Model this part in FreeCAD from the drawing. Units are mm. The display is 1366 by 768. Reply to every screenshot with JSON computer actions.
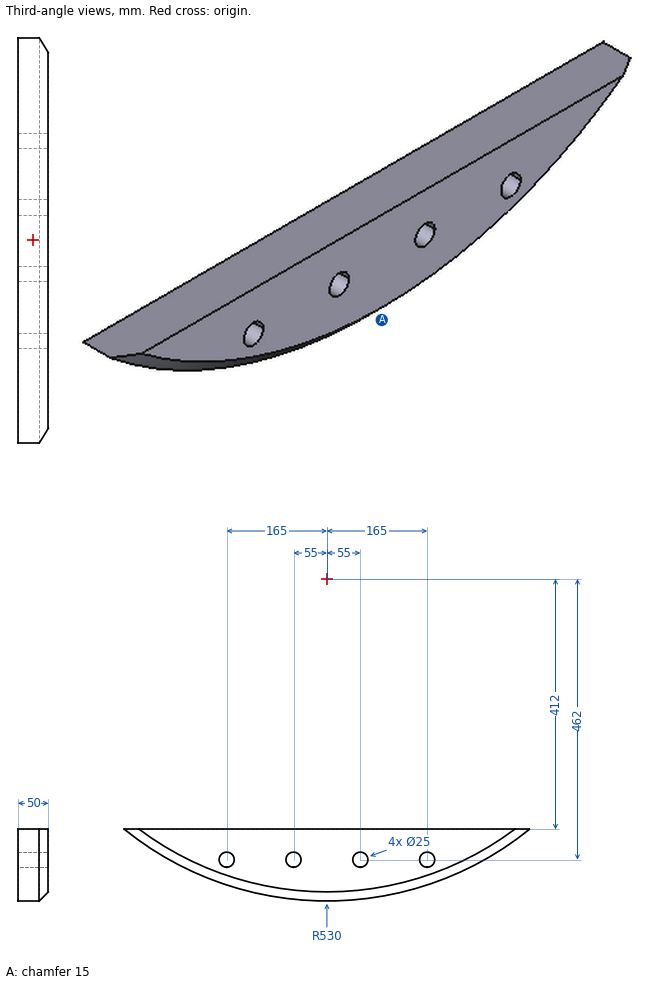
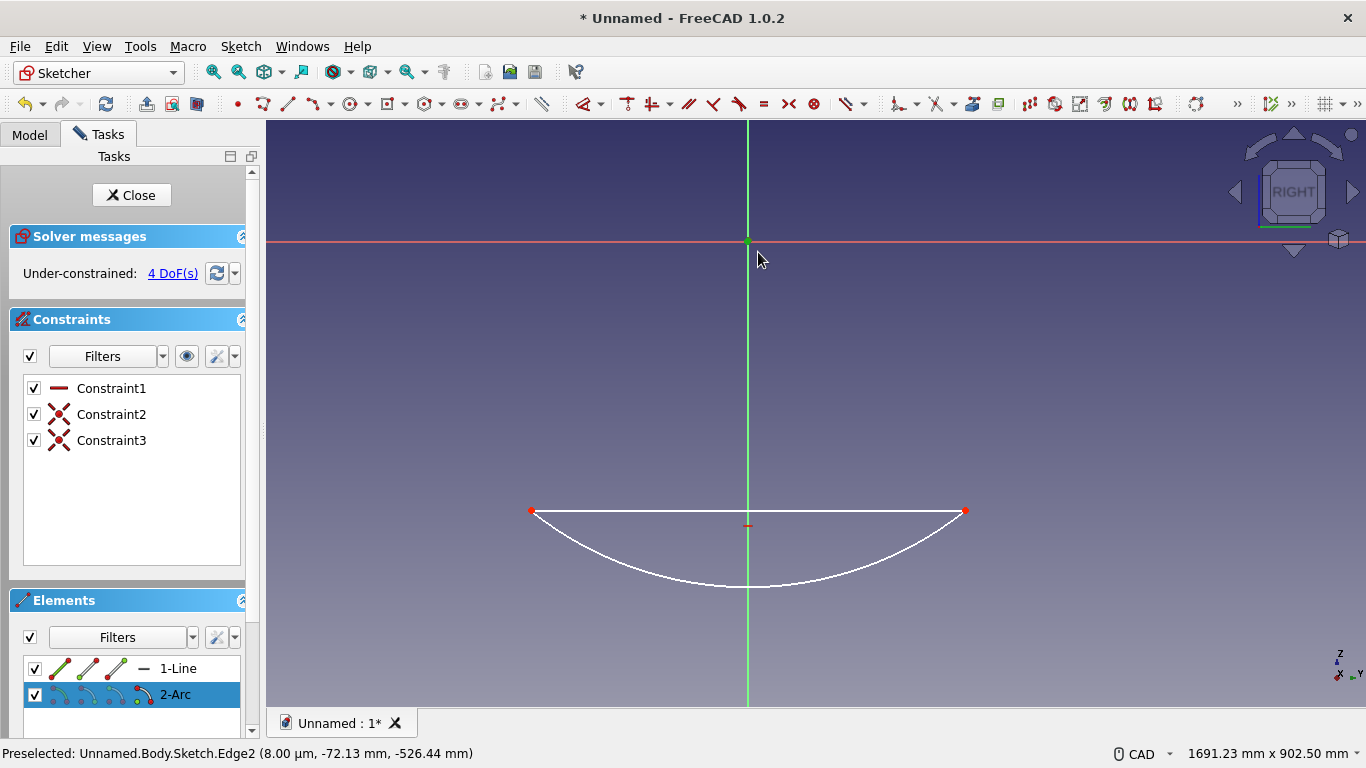
{"action": "left_click", "coordinate": [627, 104]}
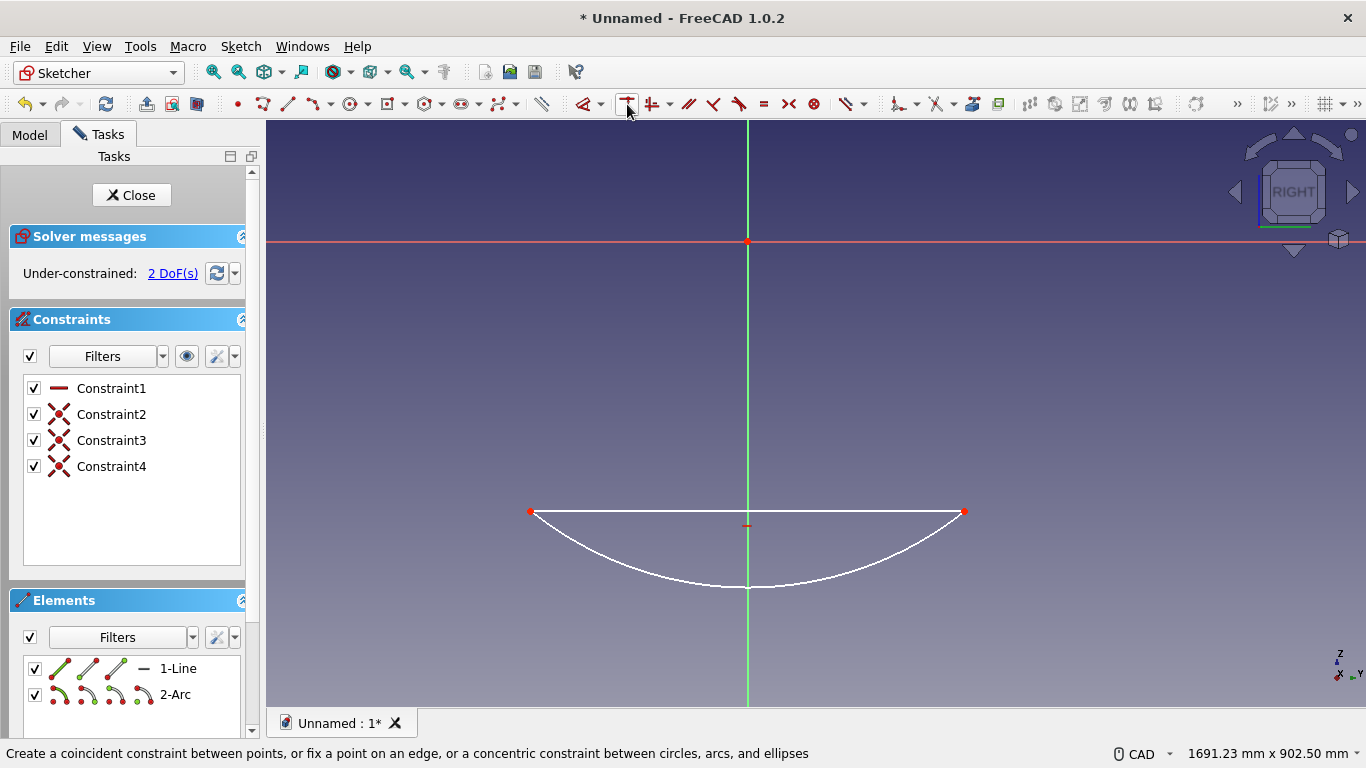
{"action": "left_click", "coordinate": [582, 104]}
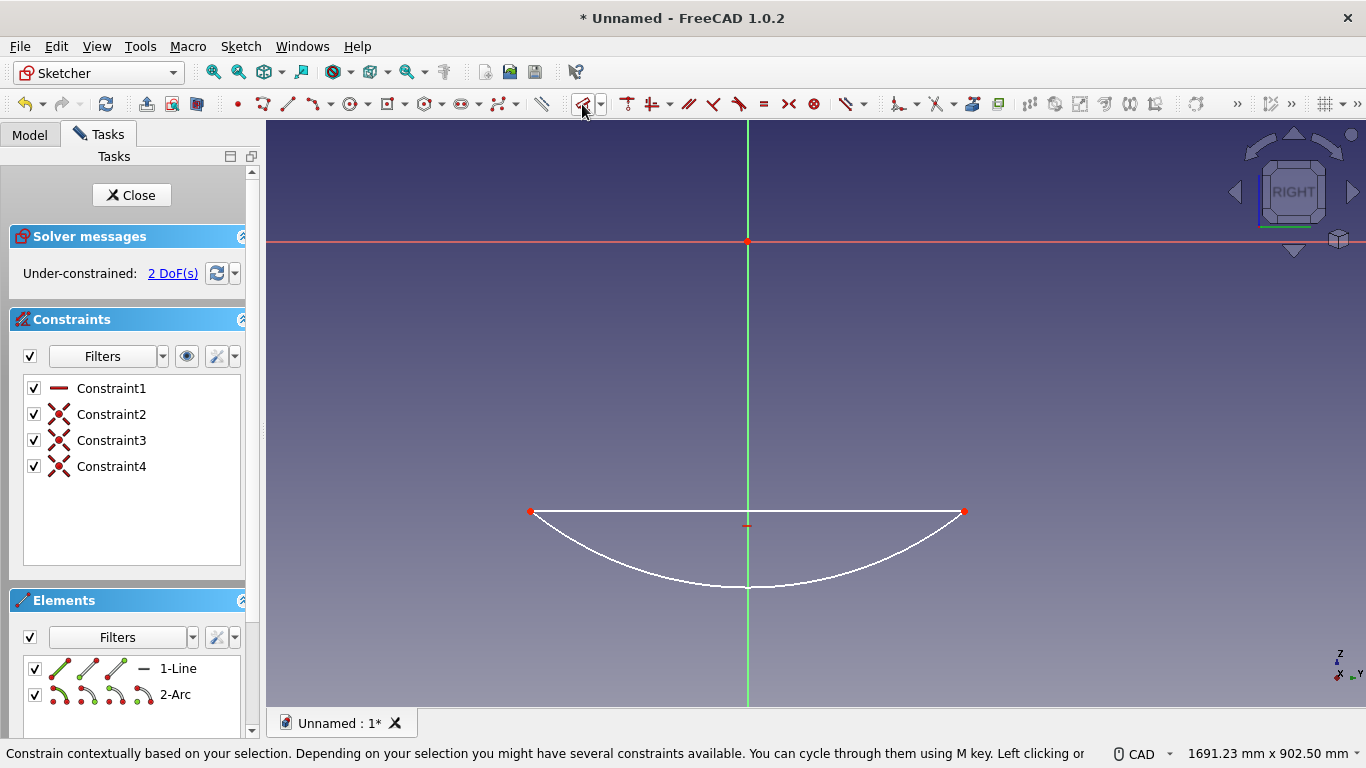
{"action": "left_click", "coordinate": [655, 575]}
{"action": "left_click", "coordinate": [646, 606]}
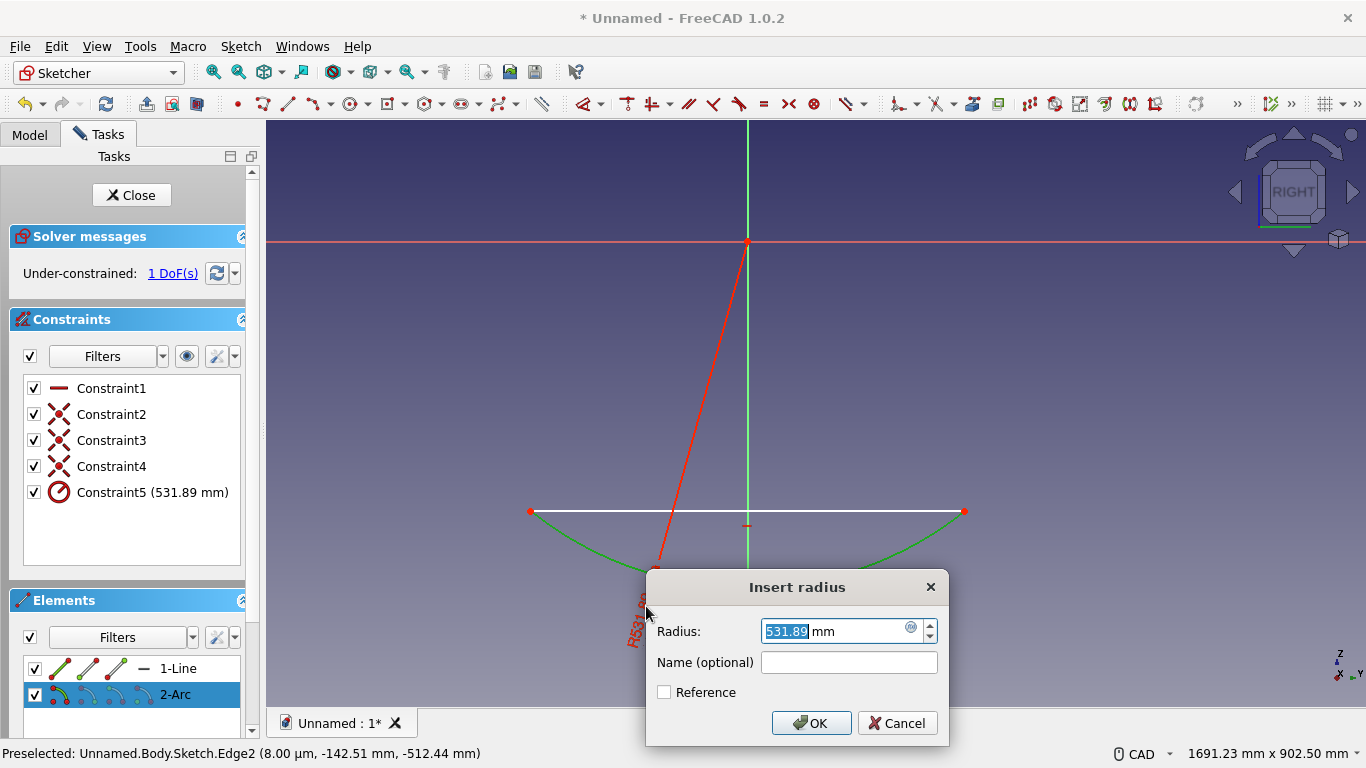
{"action": "type", "text": "530"}
{"action": "key", "text": "Return"}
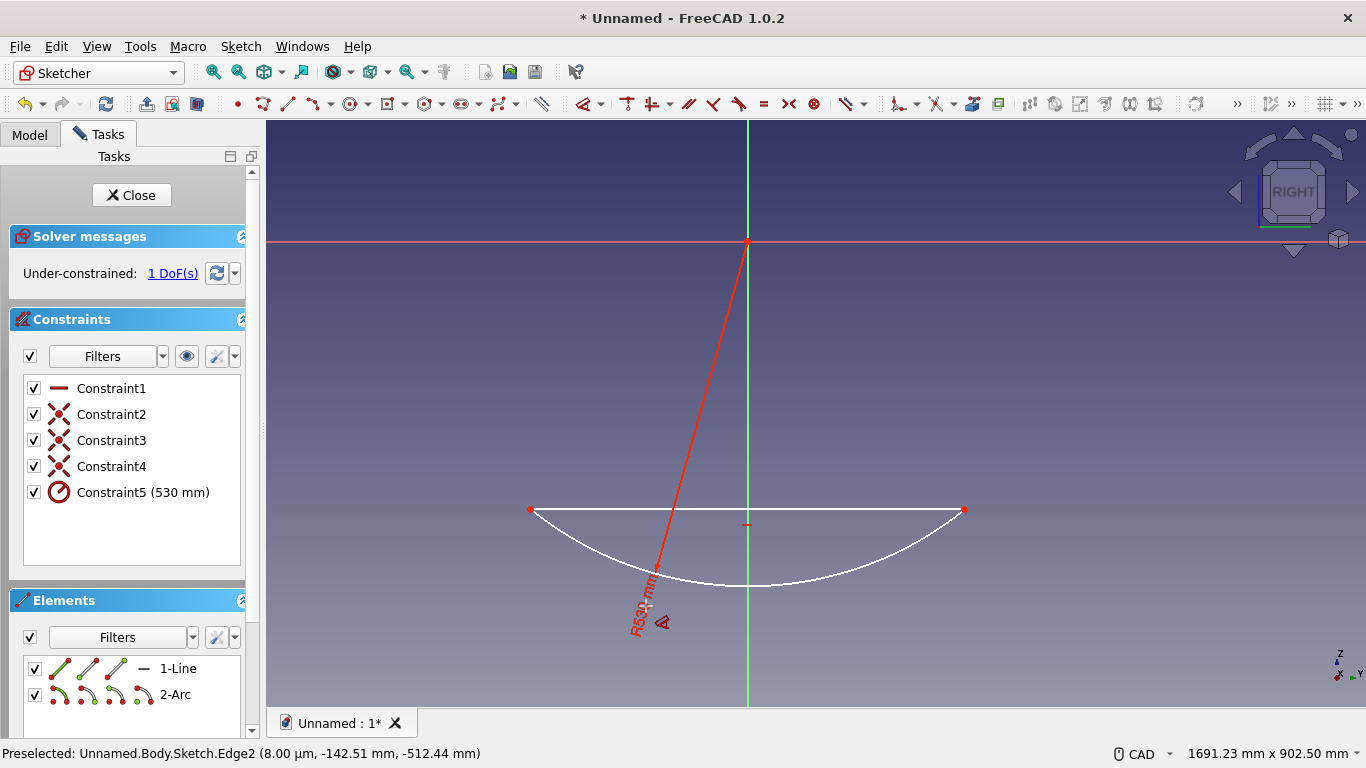
{"action": "left_click", "coordinate": [965, 509]}
{"action": "left_click", "coordinate": [999, 376]}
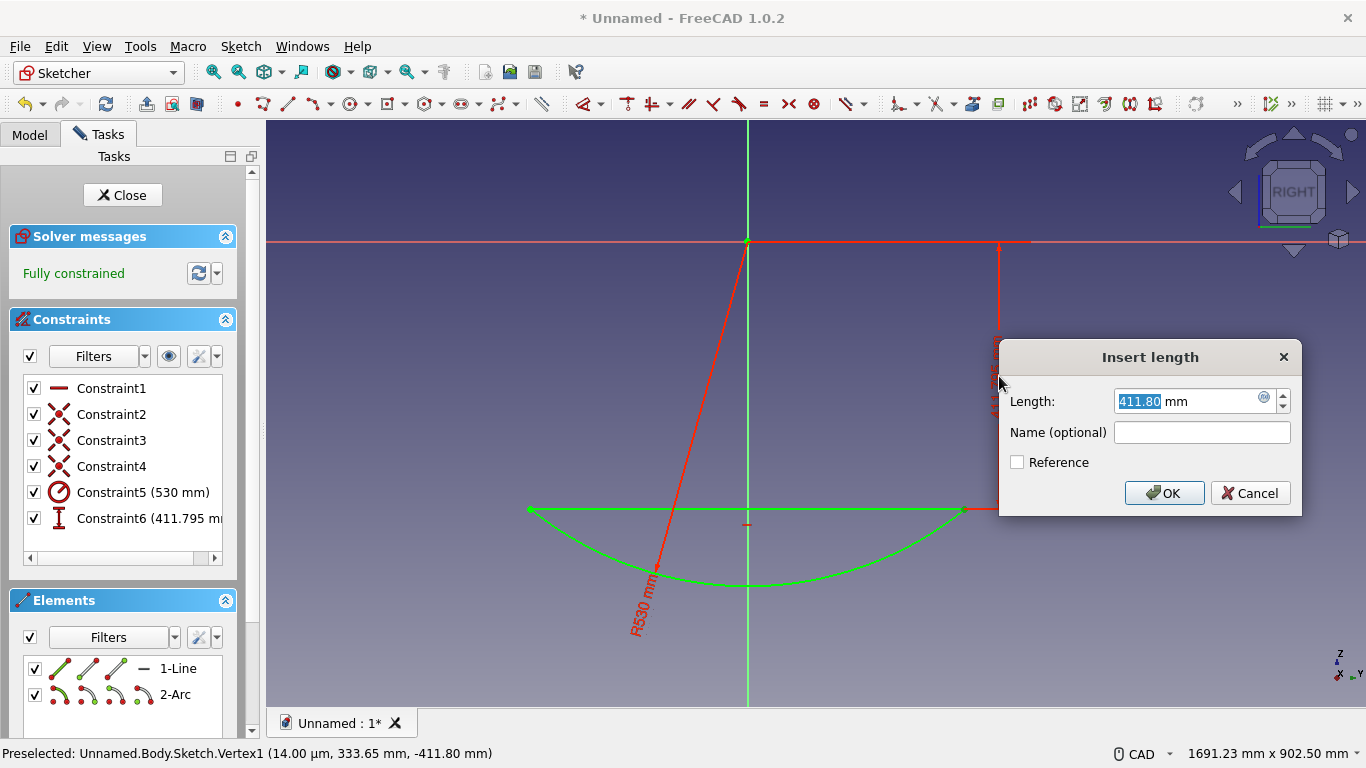
{"action": "type", "text": "412"}
{"action": "key", "text": "Return"}
{"action": "key", "text": "Escape"}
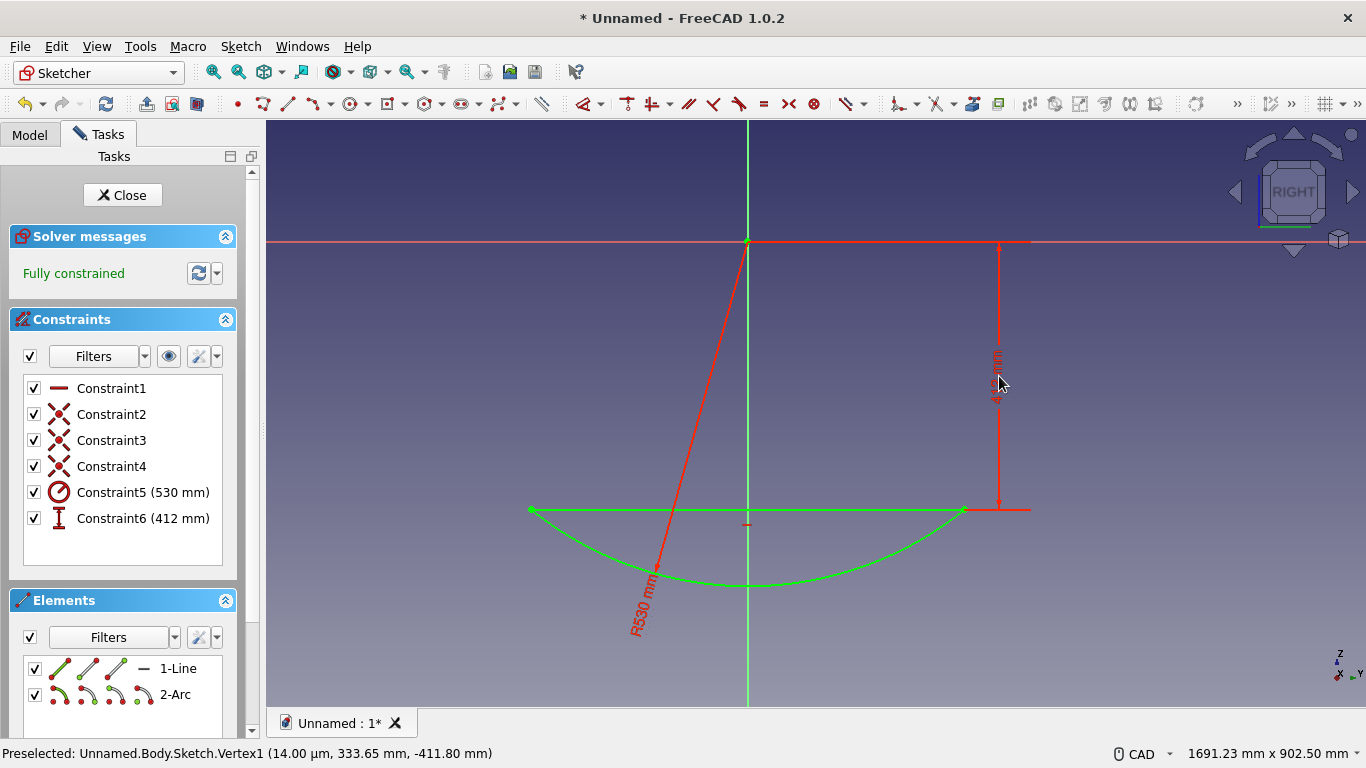
{"action": "left_click", "coordinate": [123, 195]}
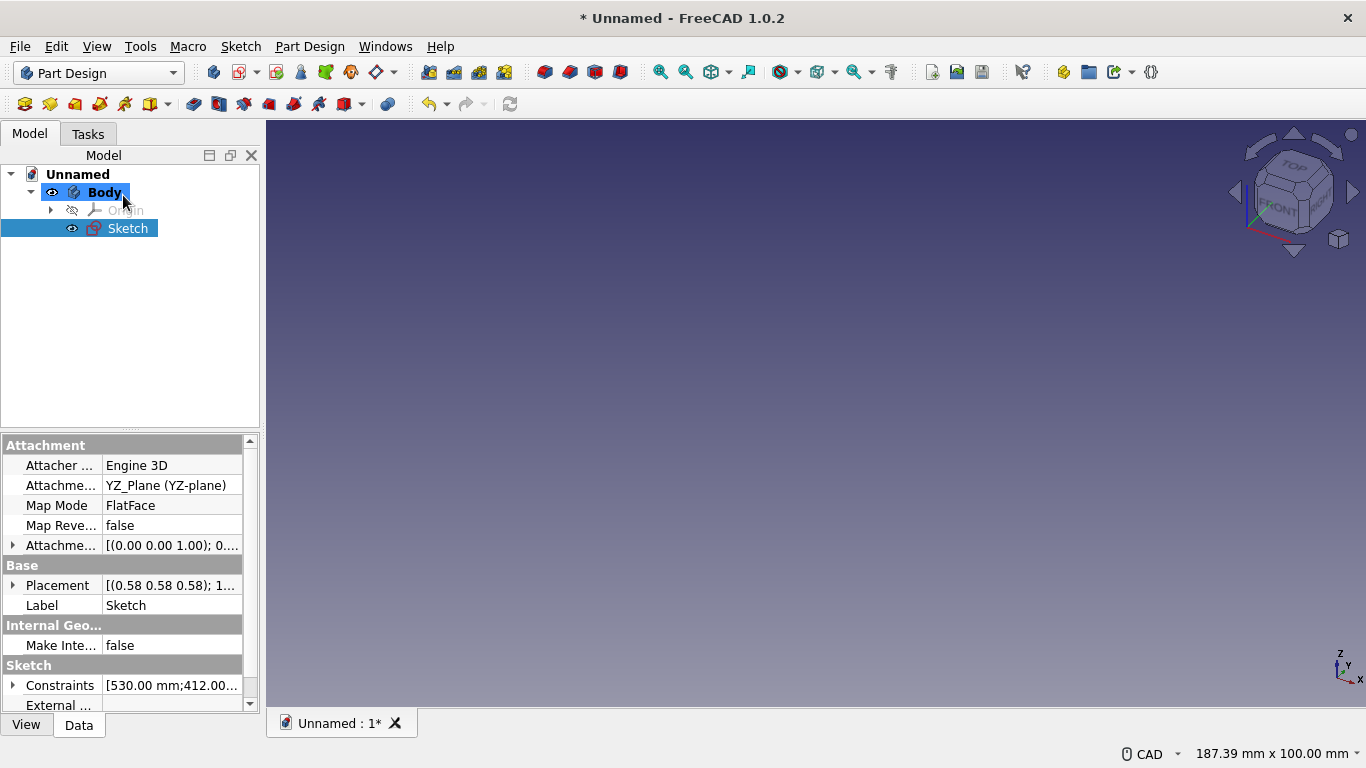
{"action": "left_click", "coordinate": [25, 104]}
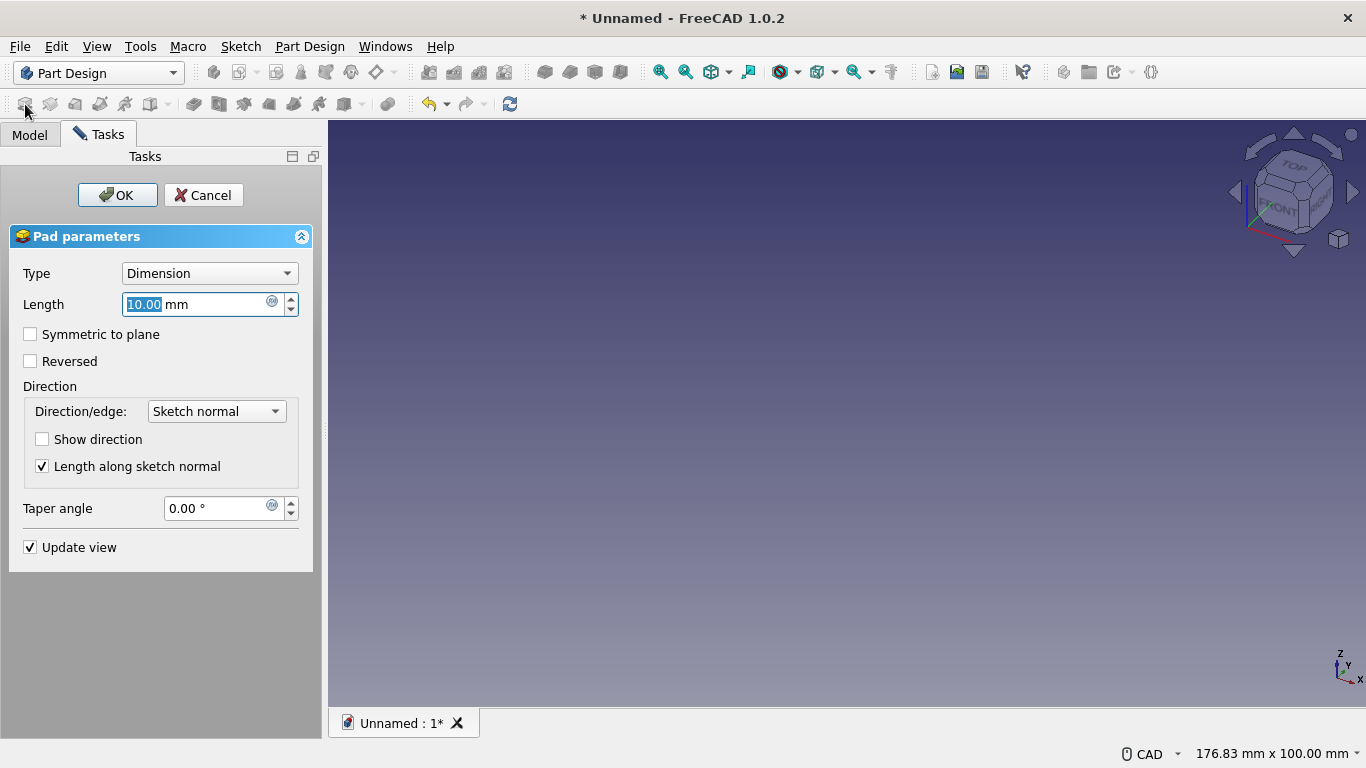
{"action": "type", "text": "50"}
{"action": "key", "text": "Tab"}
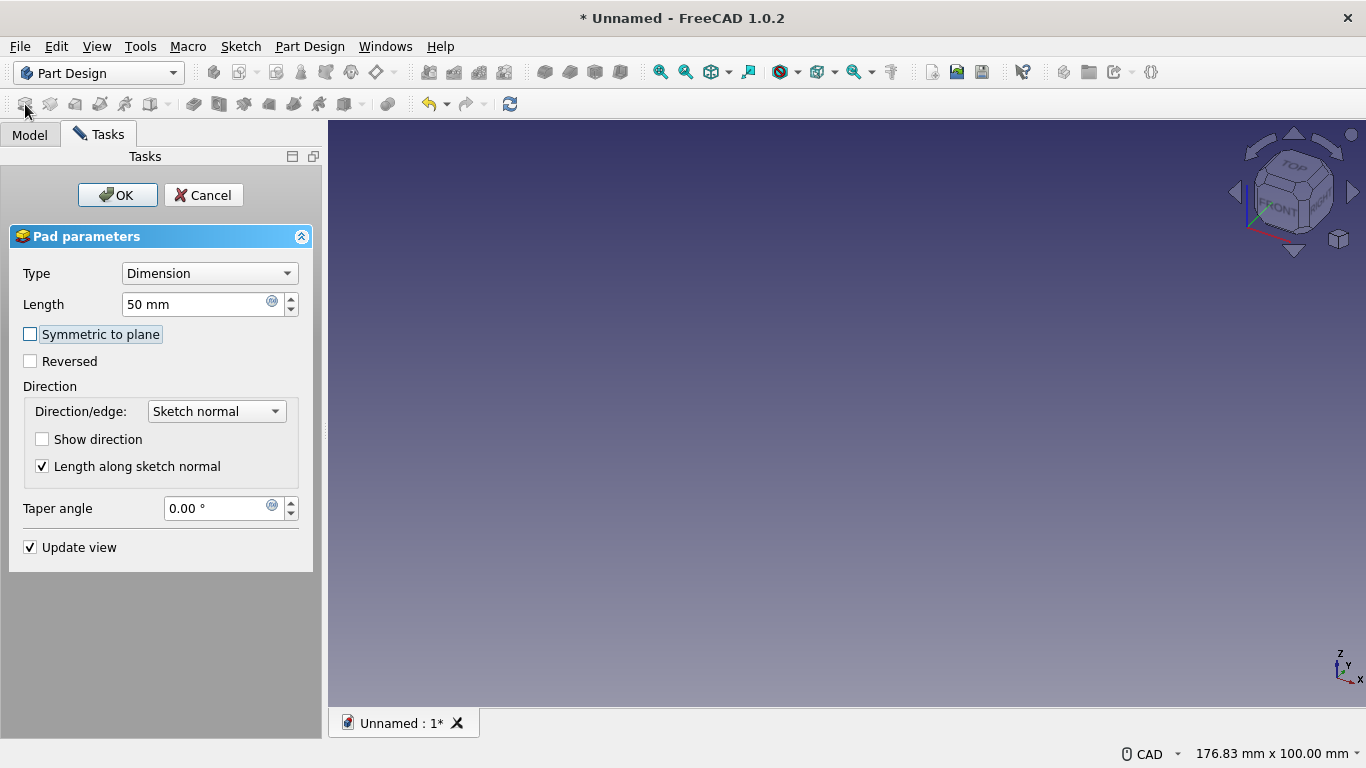
{"action": "left_click", "coordinate": [31, 334]}